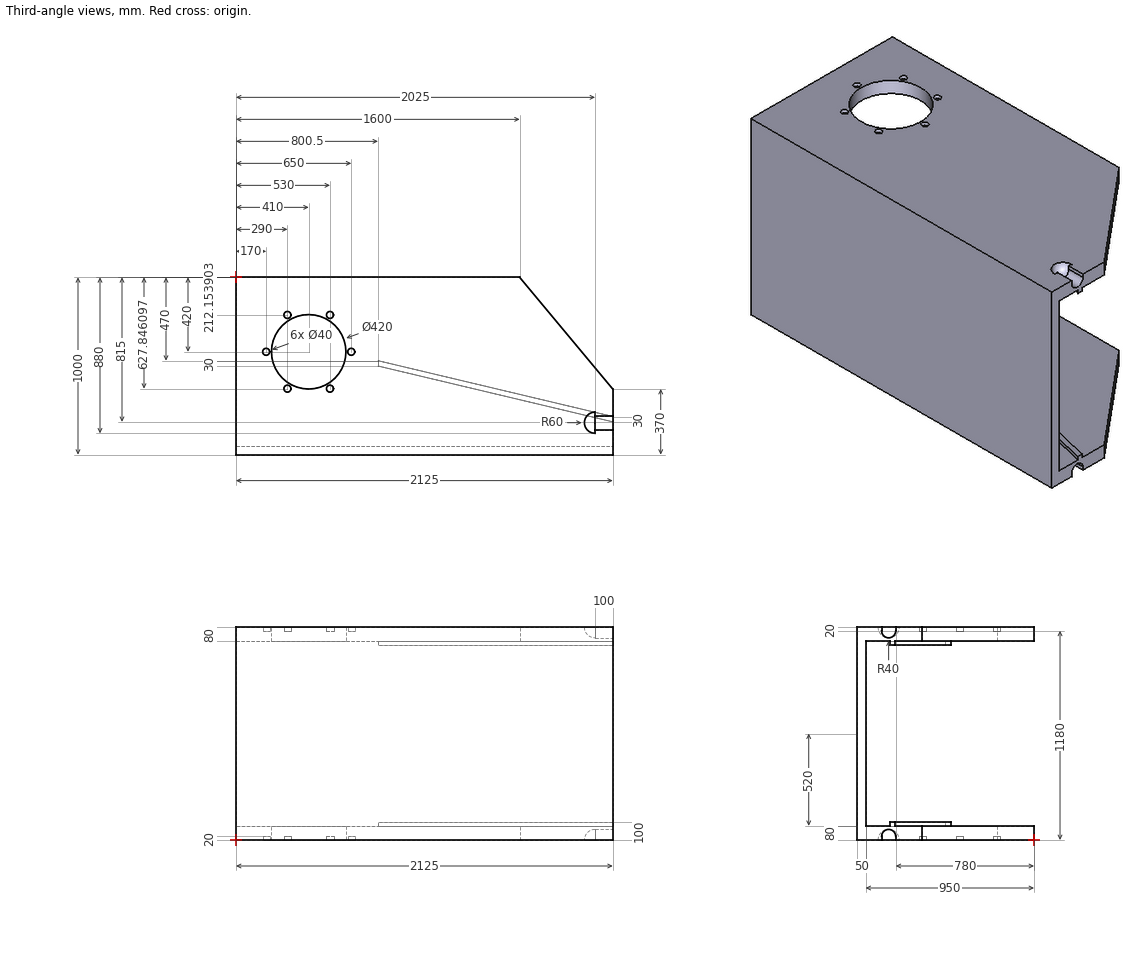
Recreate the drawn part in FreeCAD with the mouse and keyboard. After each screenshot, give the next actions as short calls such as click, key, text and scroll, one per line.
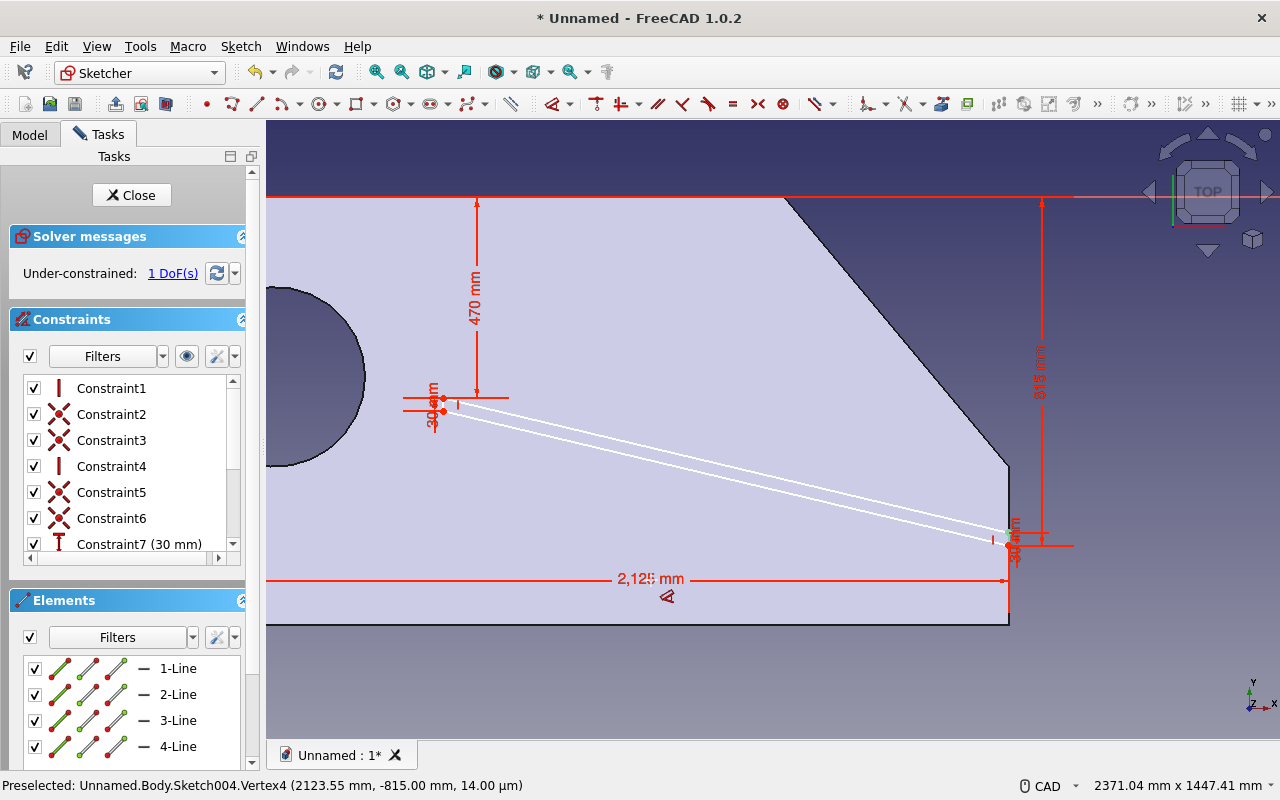
click(443, 398)
click(369, 163)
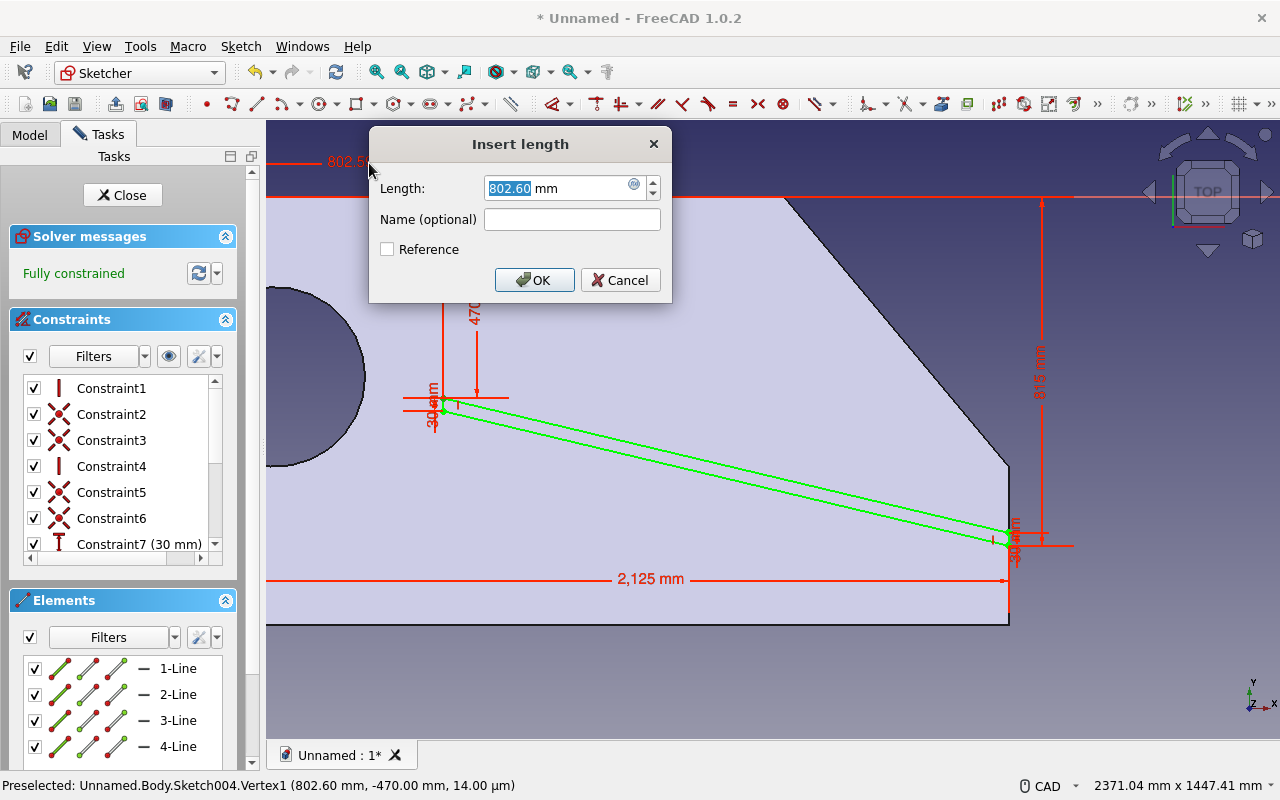
text(800.5)
key(Return)
key(Escape)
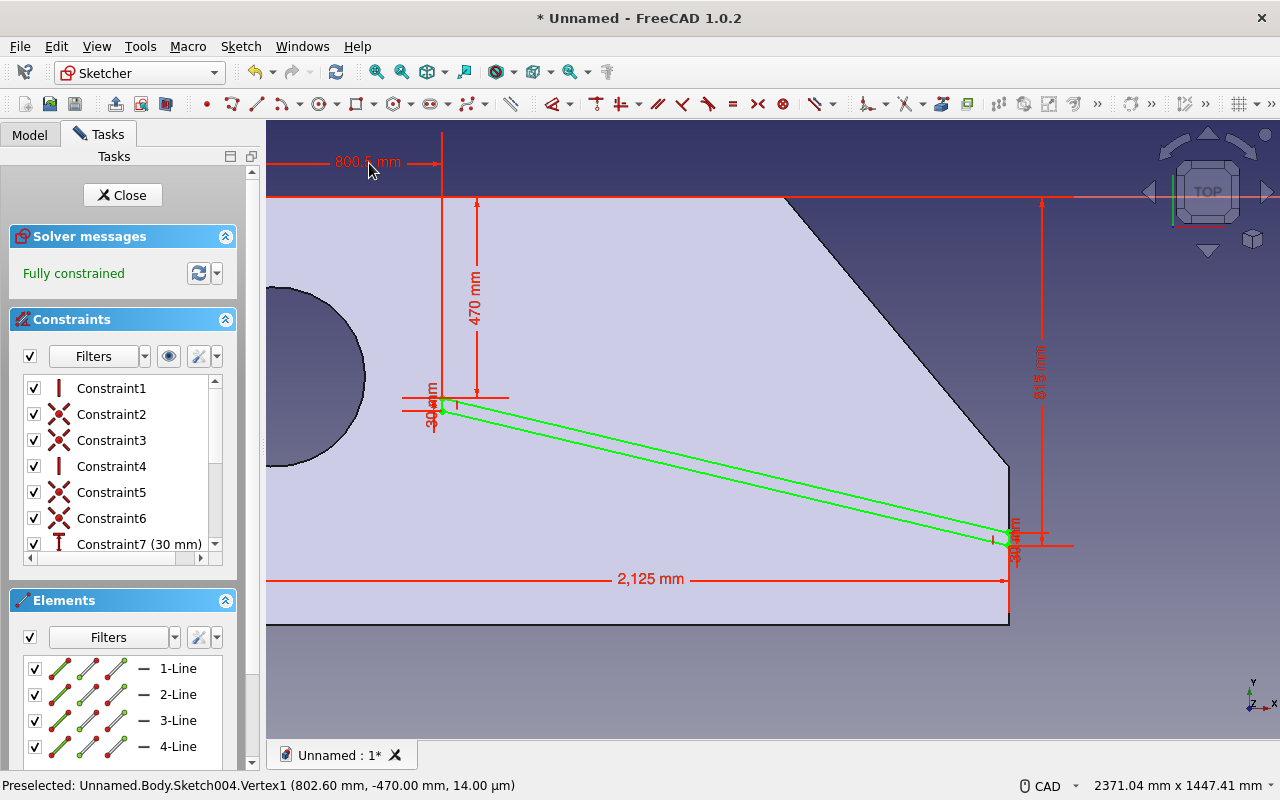
click(123, 195)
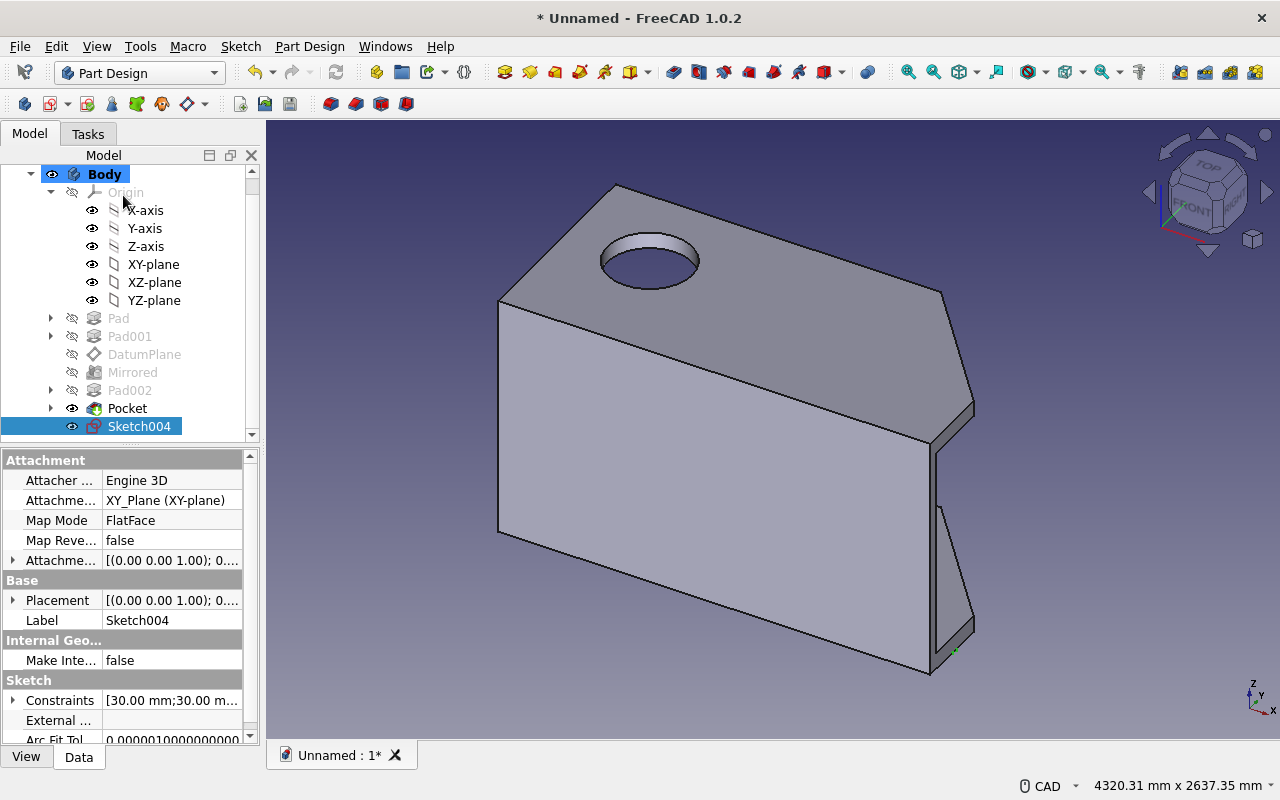
click(505, 72)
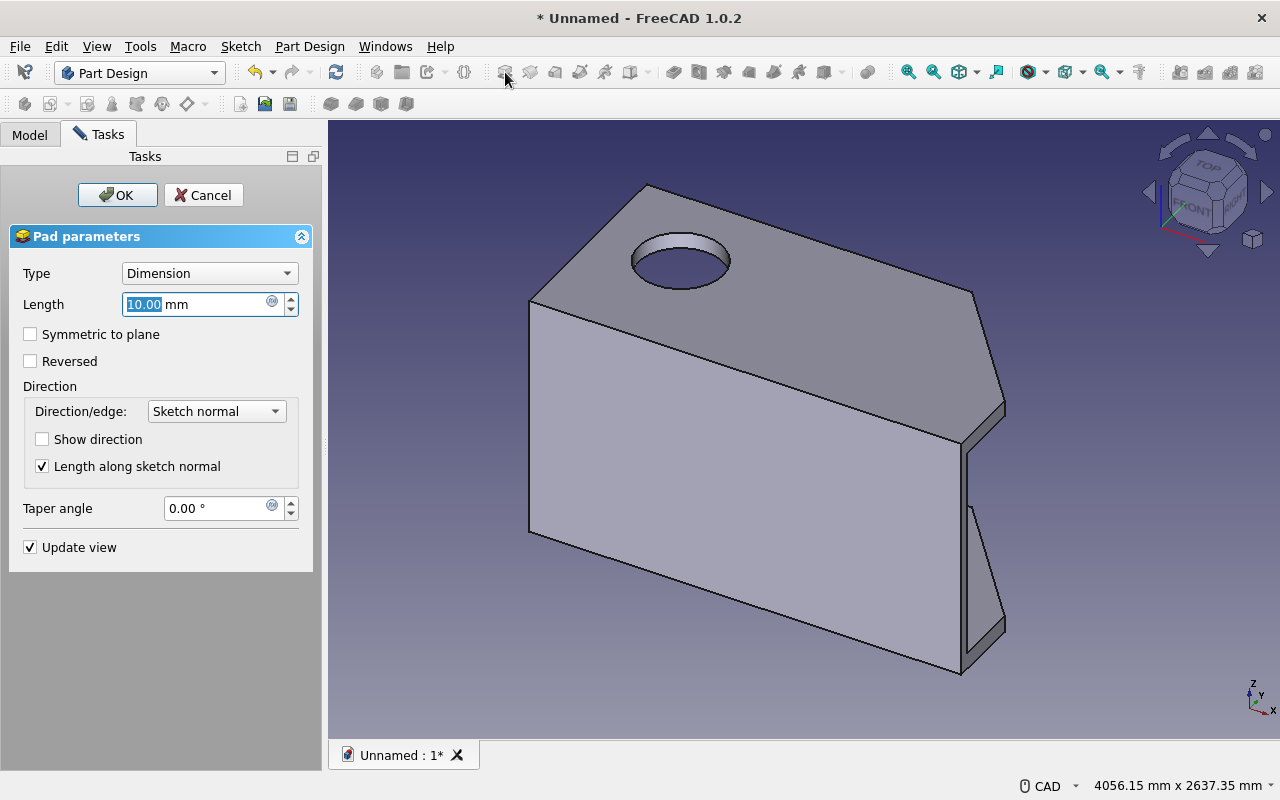
text(100)
key(Tab)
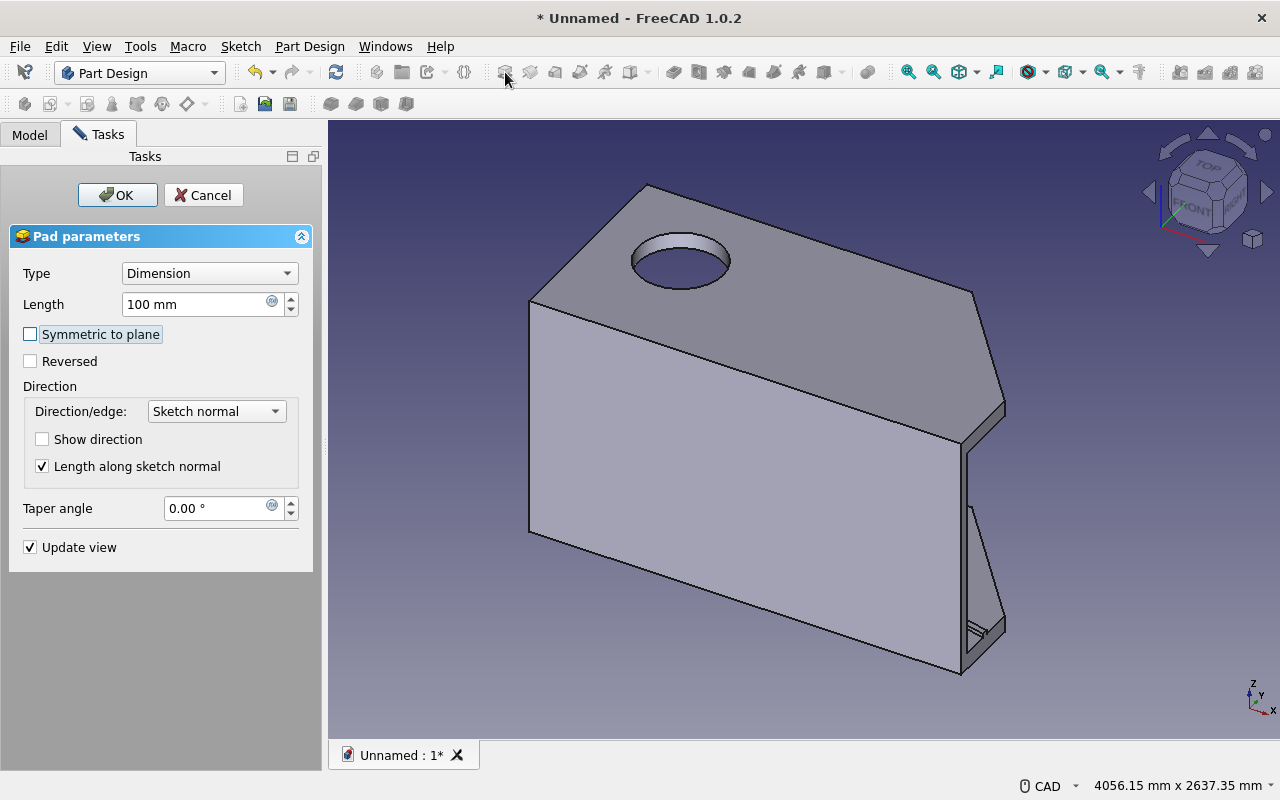
click(118, 195)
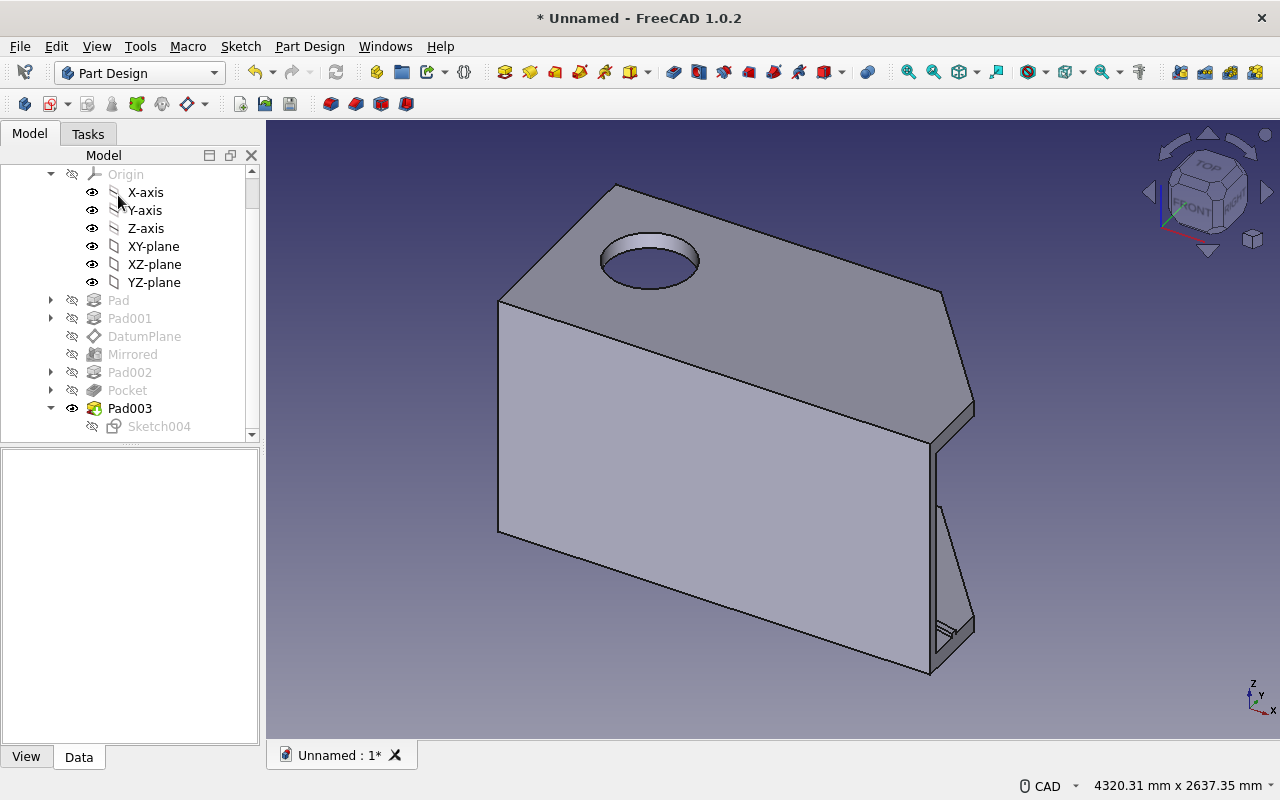
click(137, 246)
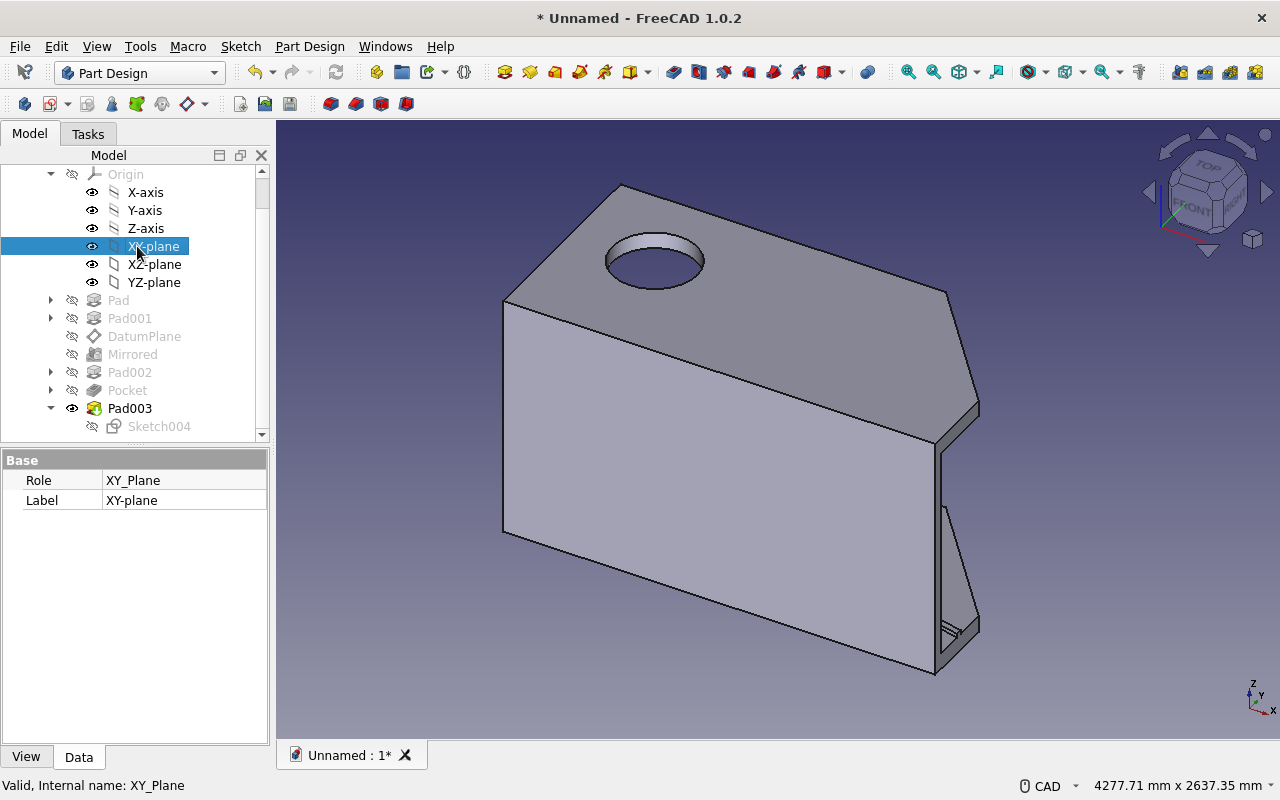
click(186, 104)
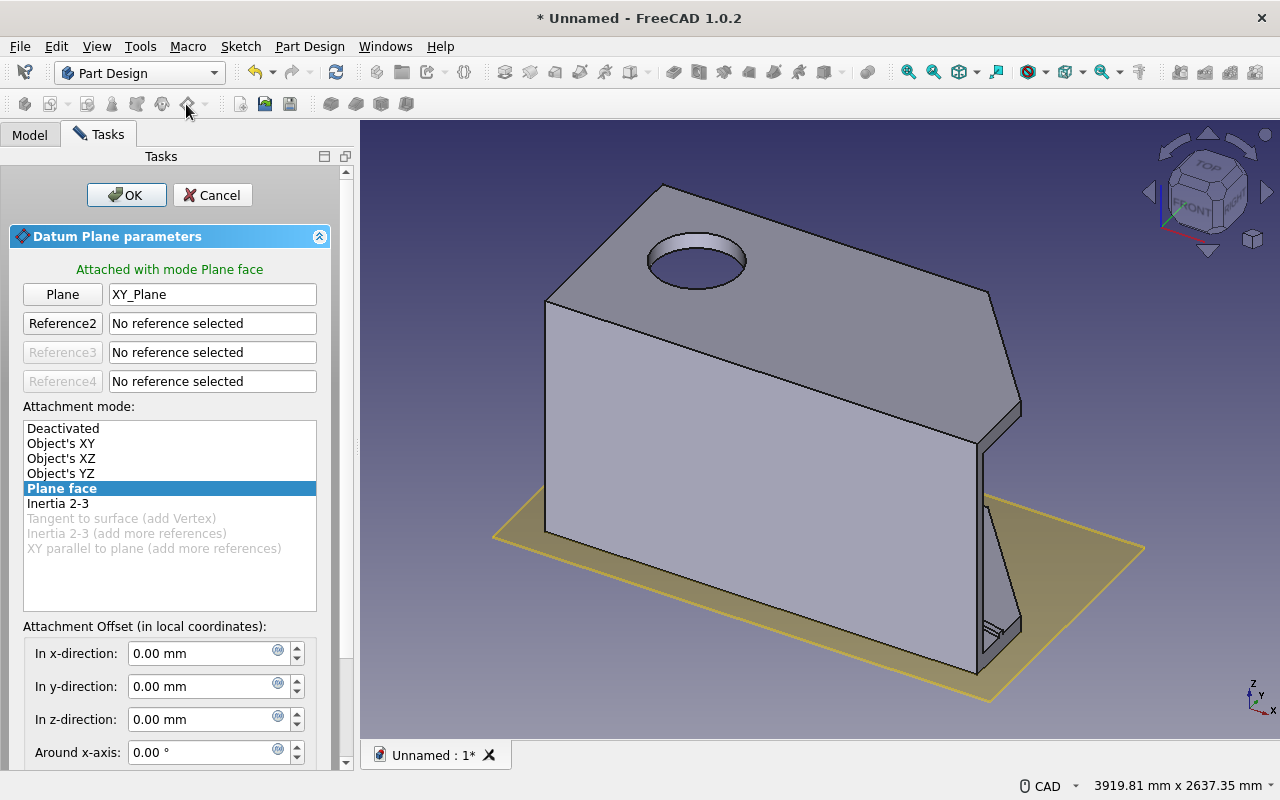
triple_click(210, 720)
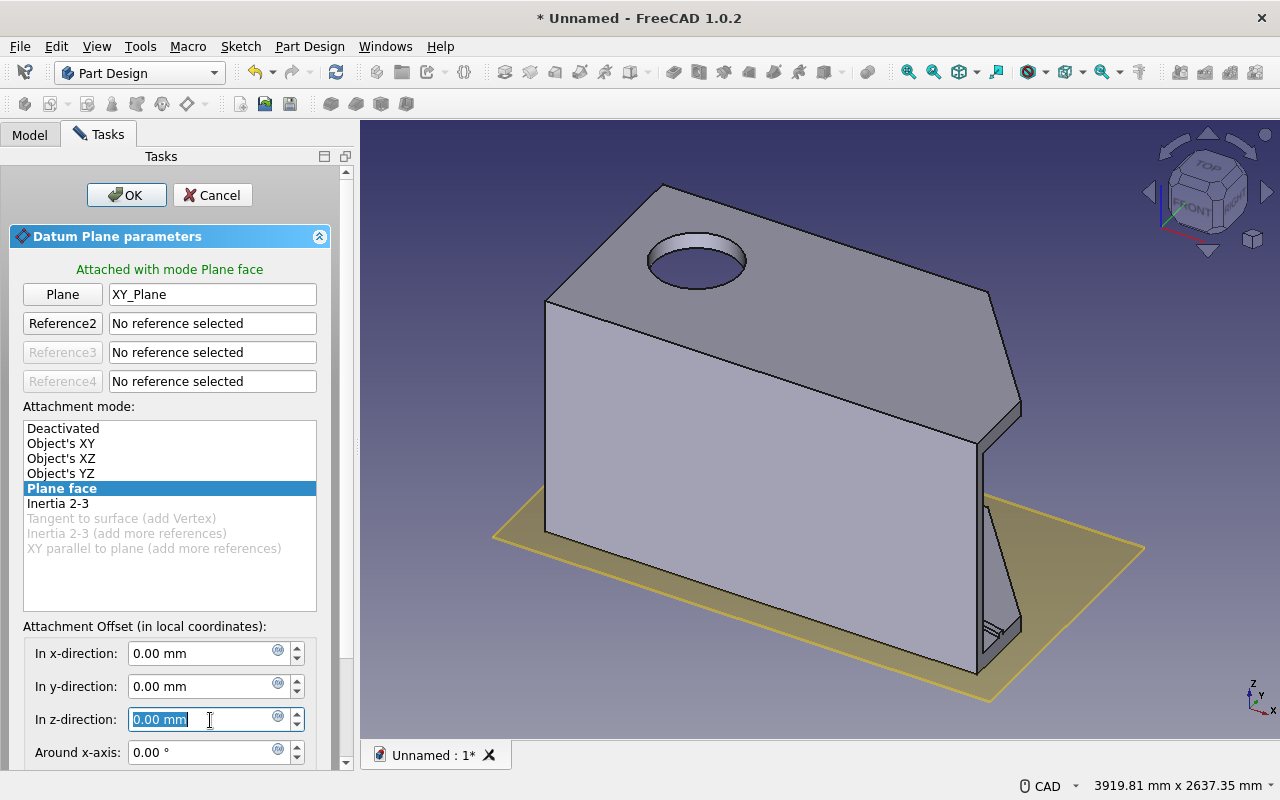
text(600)
key(Tab)